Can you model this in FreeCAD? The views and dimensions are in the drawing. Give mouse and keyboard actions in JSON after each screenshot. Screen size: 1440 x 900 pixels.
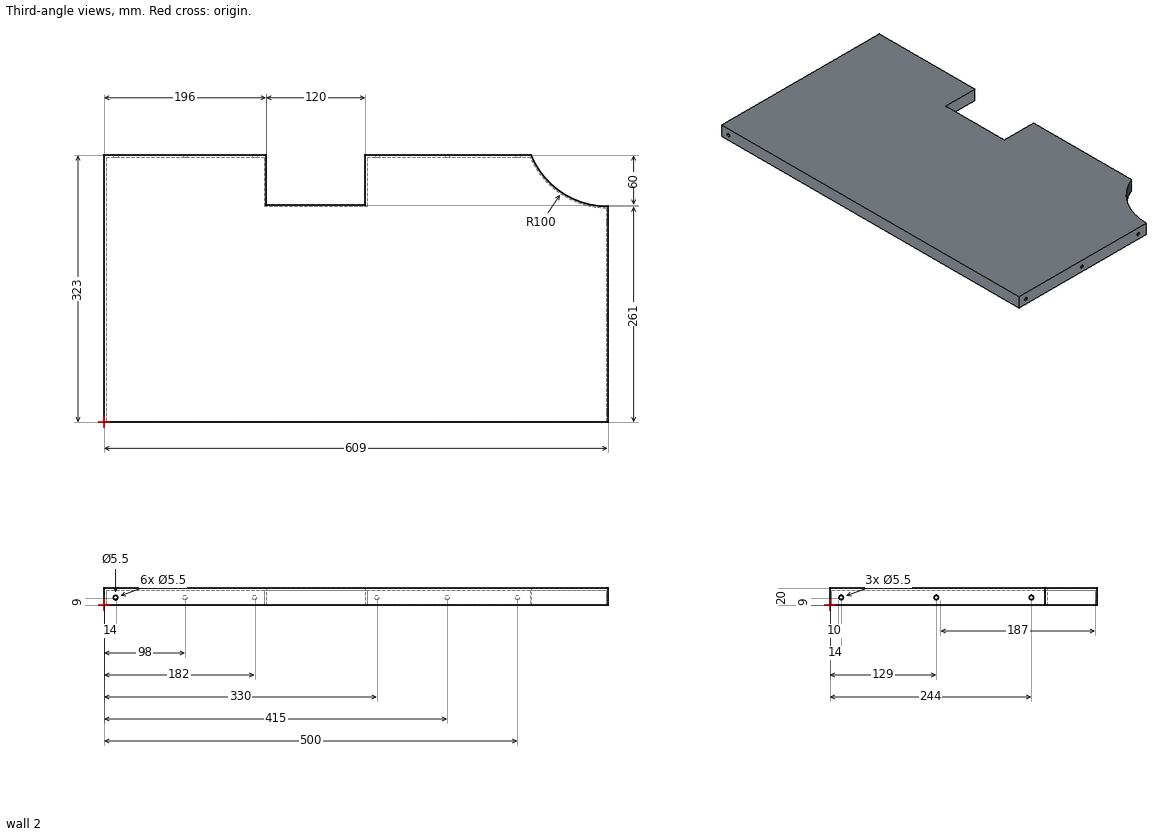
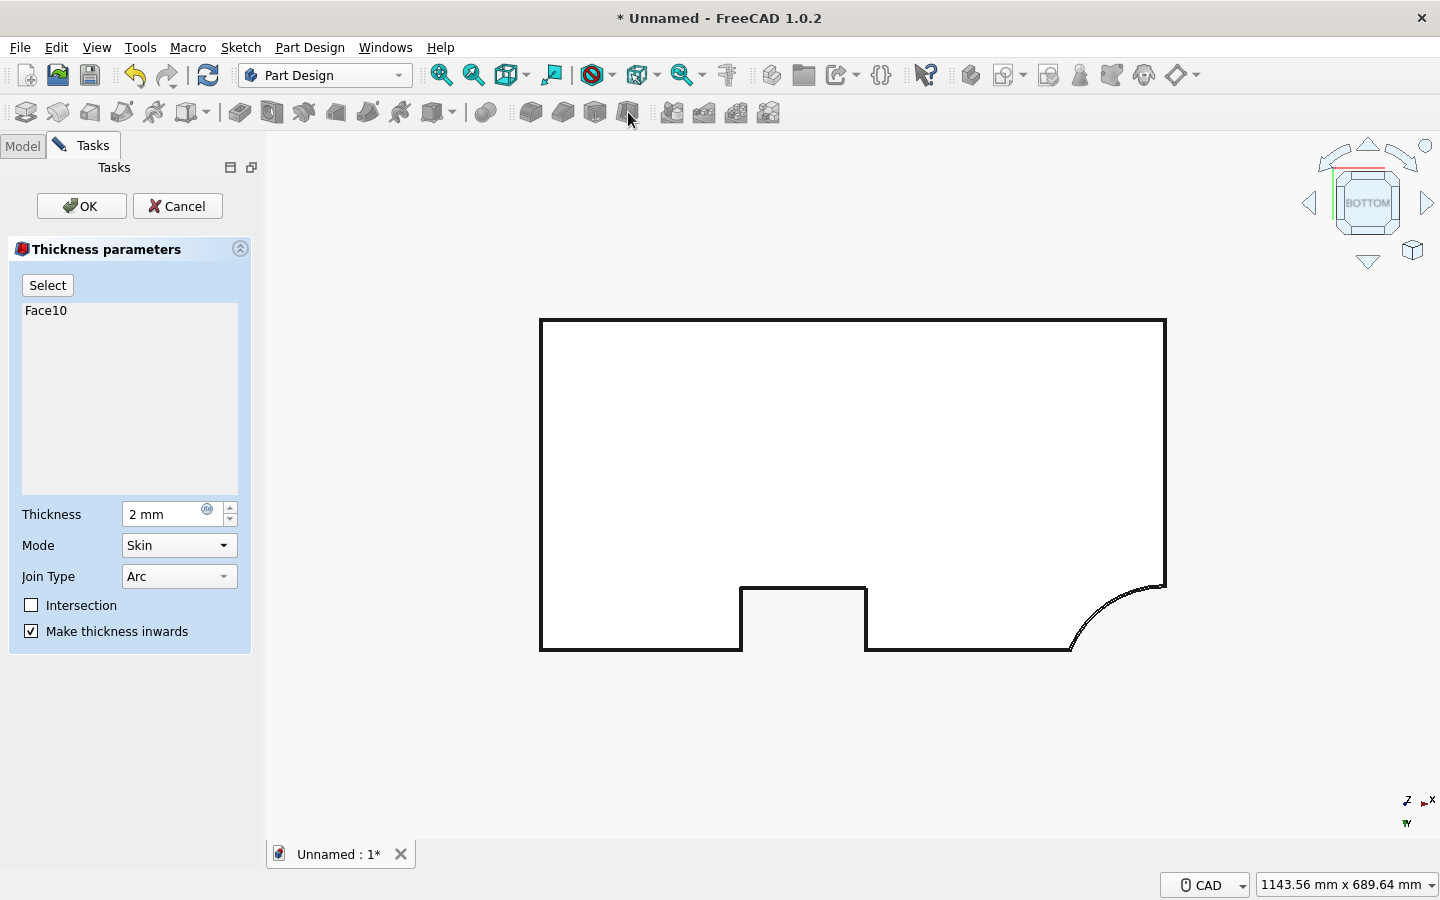
{"action": "left_click", "coordinate": [180, 576]}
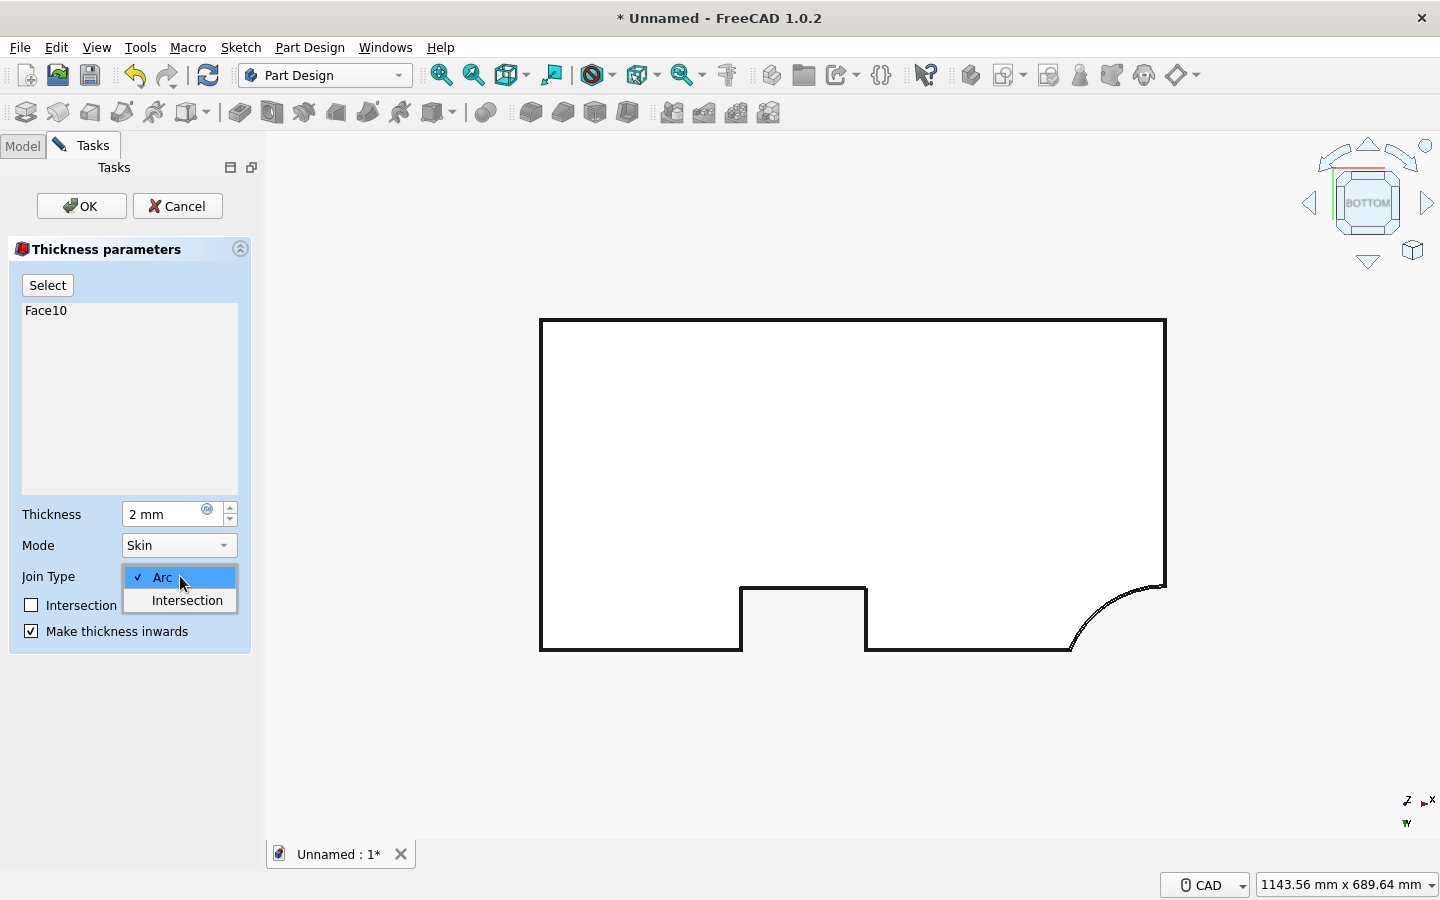
{"action": "left_click", "coordinate": [179, 600]}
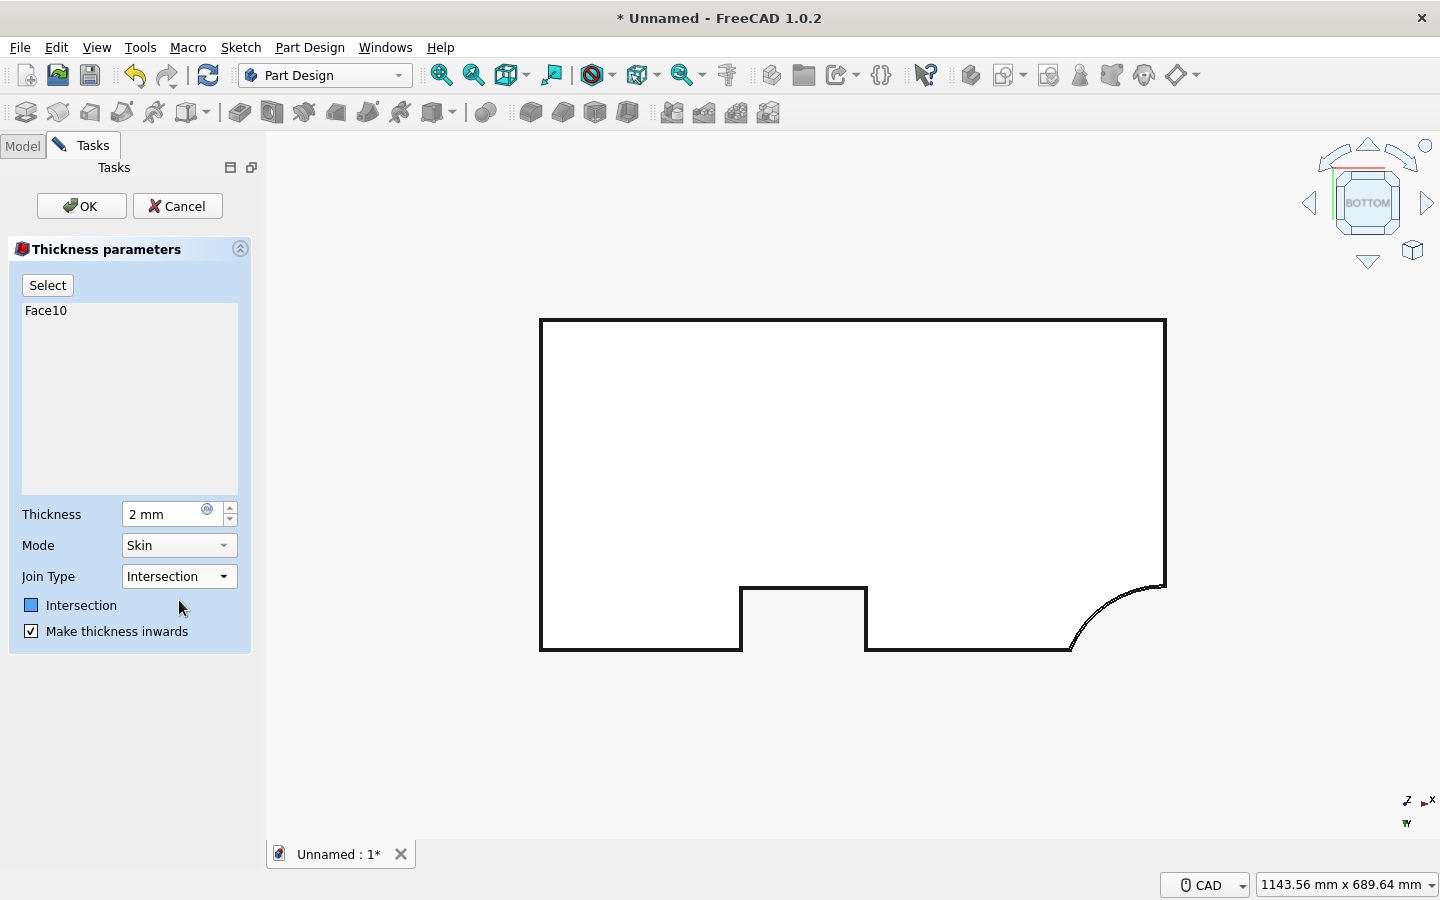
{"action": "left_click", "coordinate": [82, 206]}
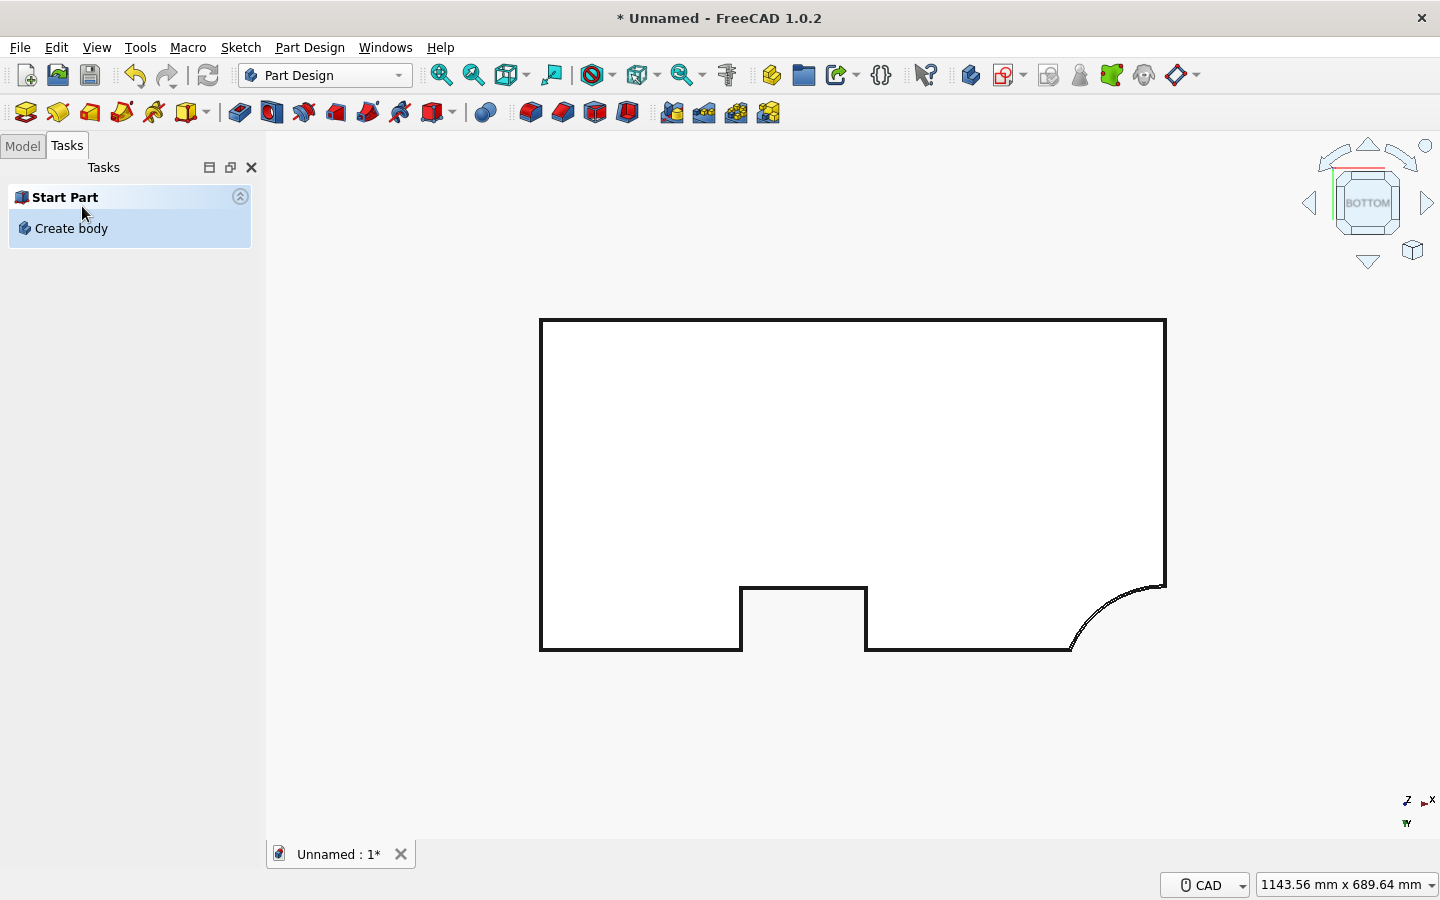
{"action": "left_click", "coordinate": [23, 145]}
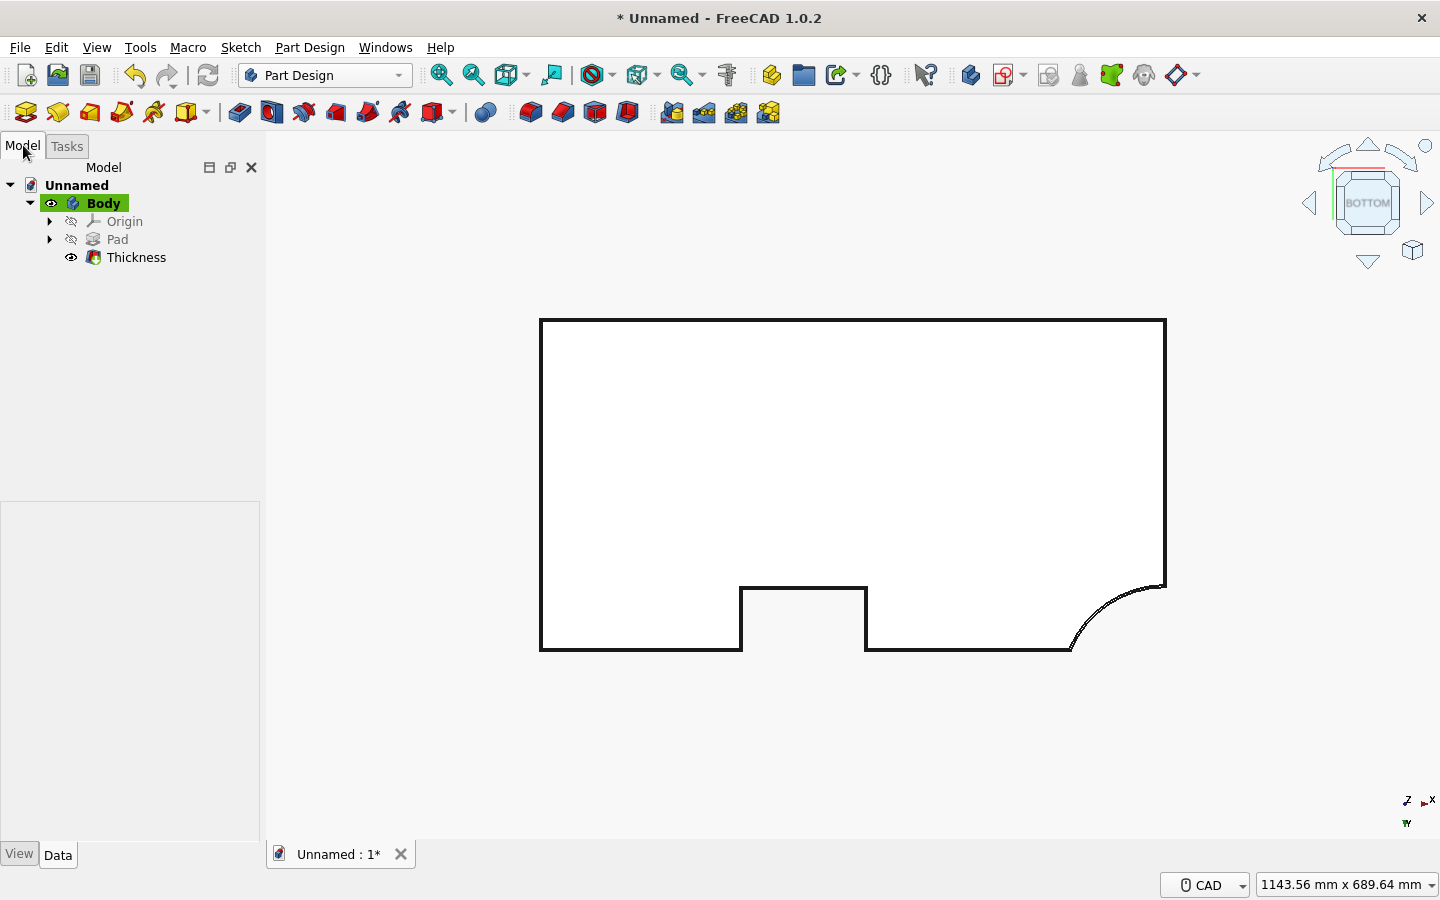
{"action": "left_click", "coordinate": [50, 221]}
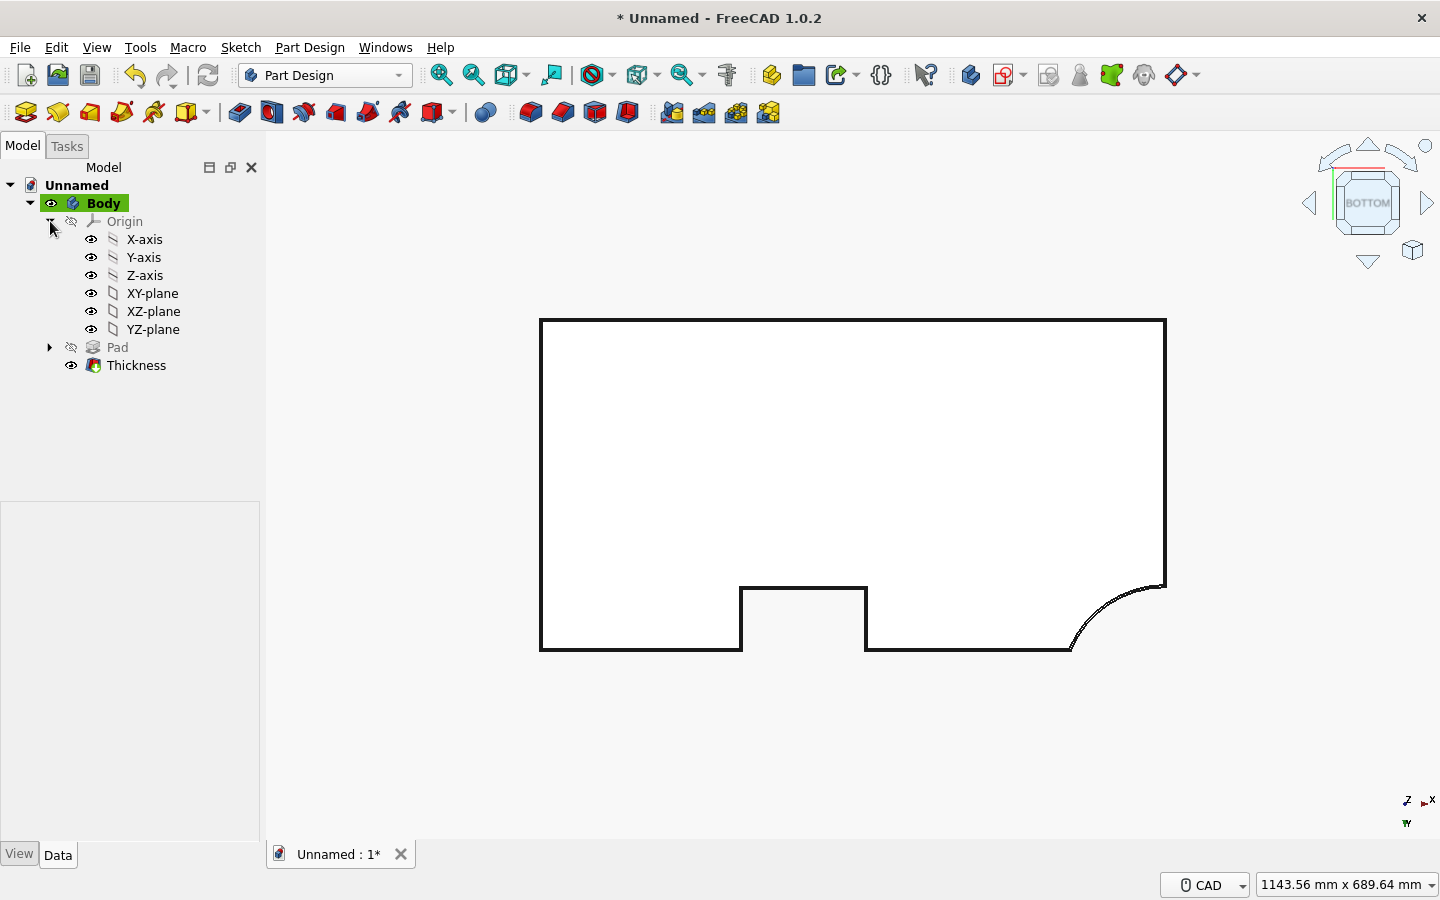
{"action": "left_click", "coordinate": [136, 311]}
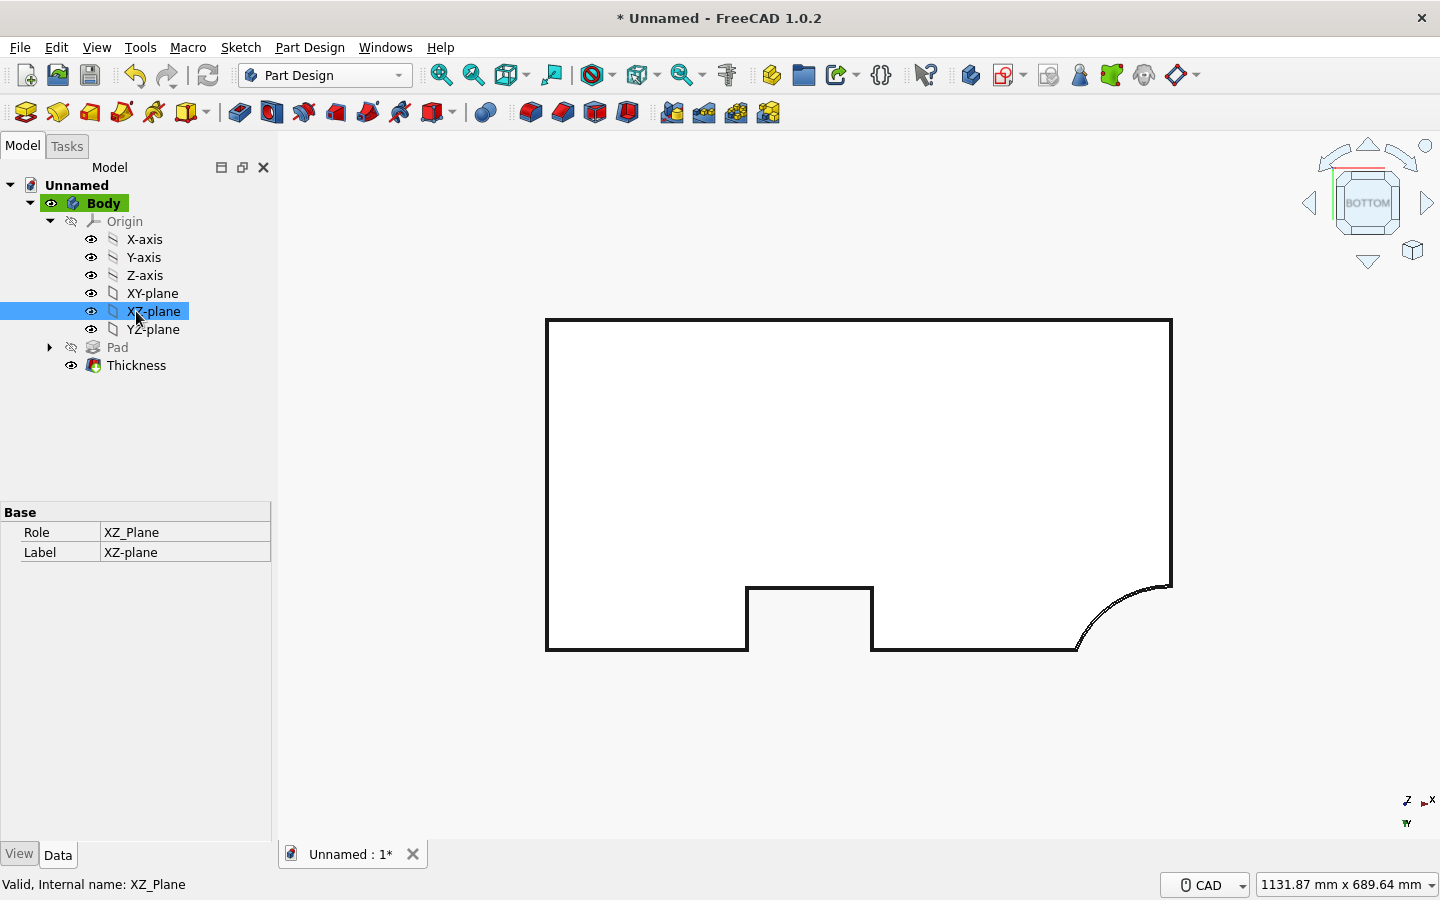
{"action": "left_click", "coordinate": [1176, 76]}